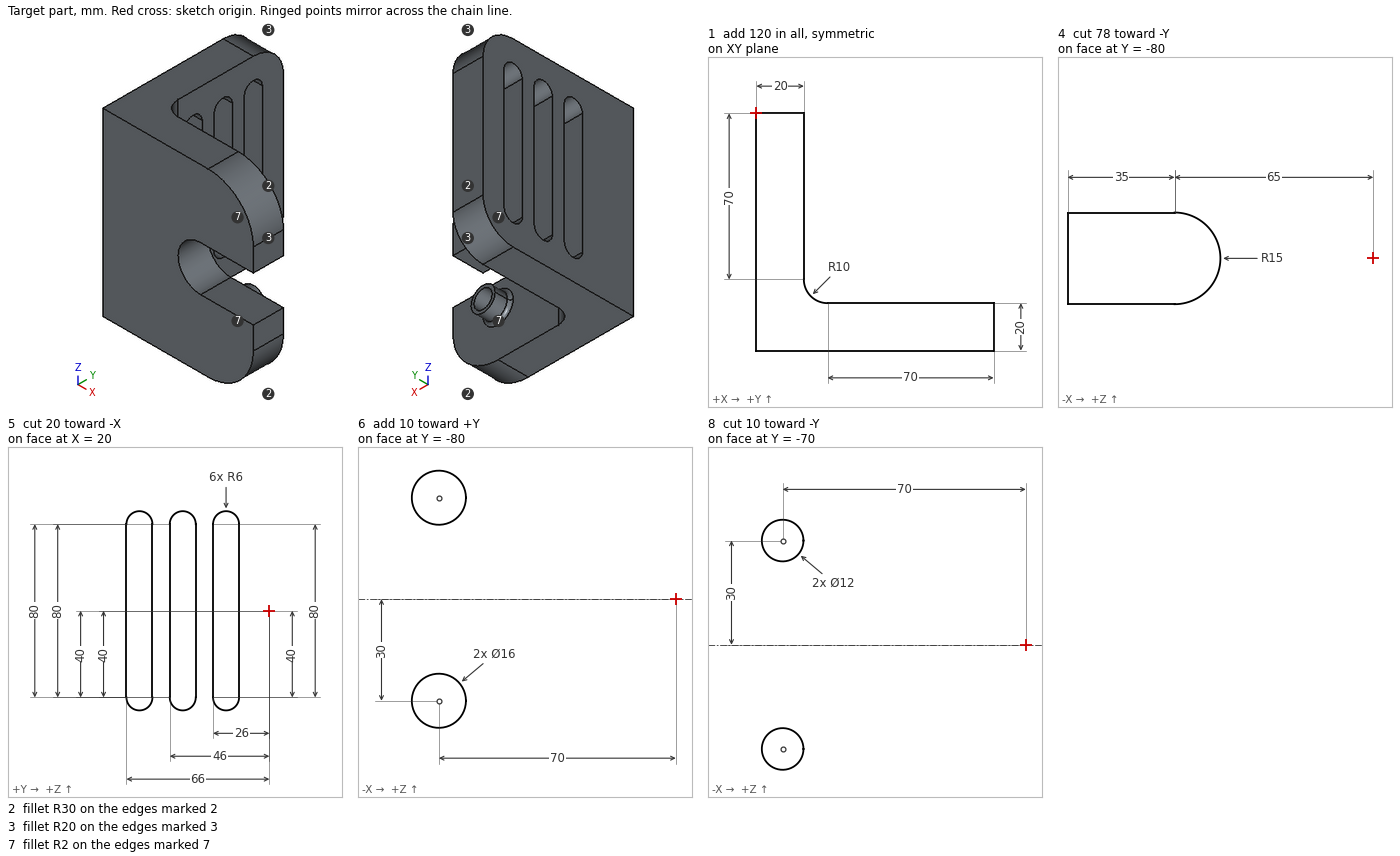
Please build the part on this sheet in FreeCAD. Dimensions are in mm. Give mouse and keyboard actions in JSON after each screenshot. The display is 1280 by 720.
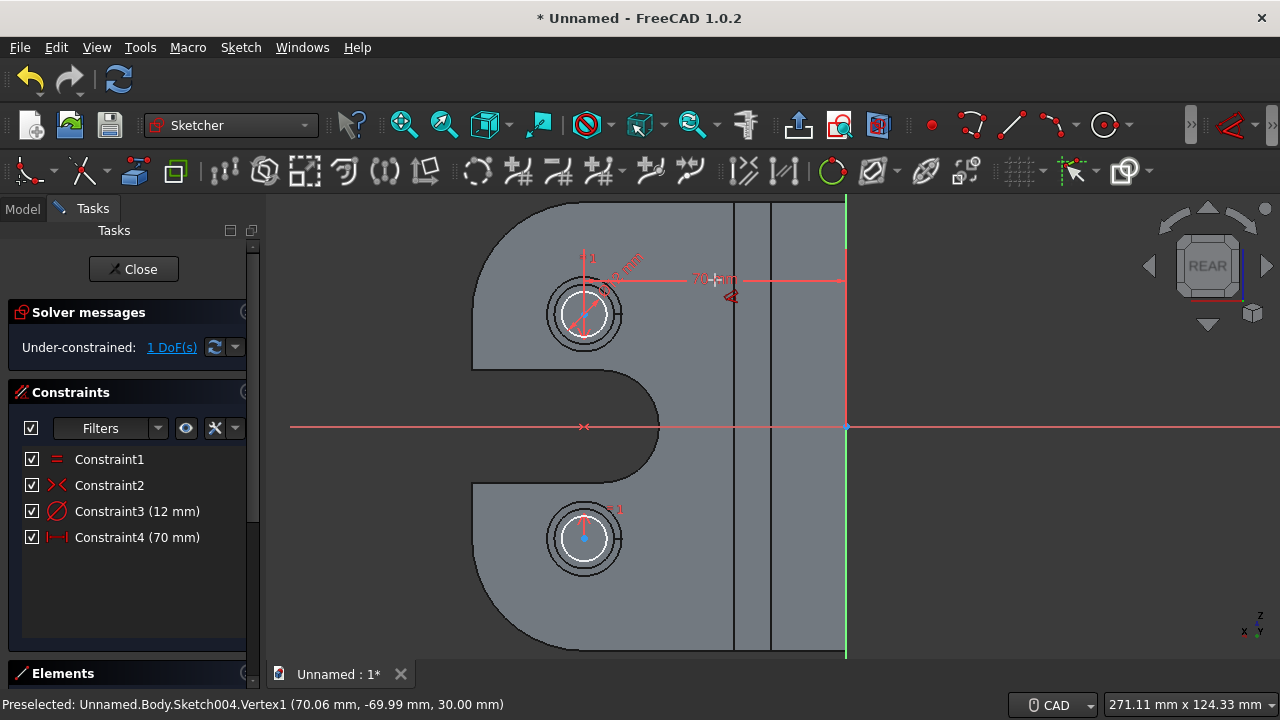
{"action": "left_click", "coordinate": [584, 314]}
{"action": "left_click", "coordinate": [880, 370]}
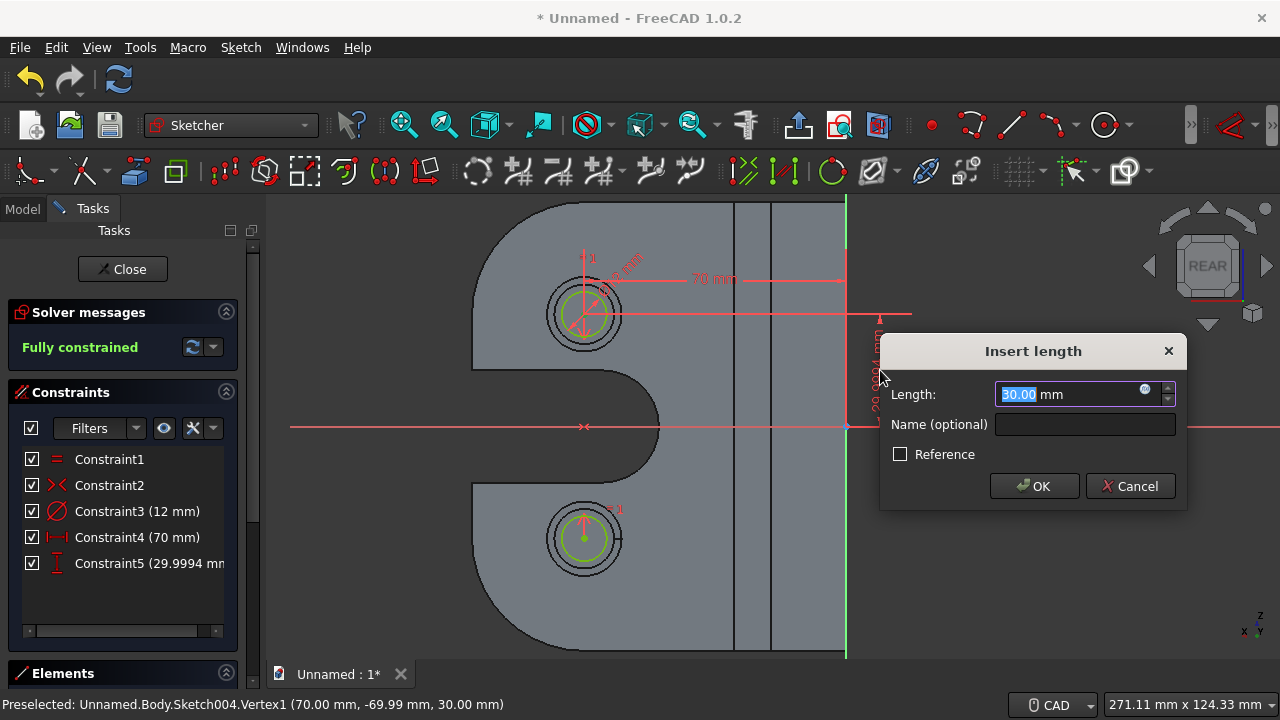
{"action": "type", "text": "30"}
{"action": "key", "text": "Return"}
{"action": "key", "text": "Escape"}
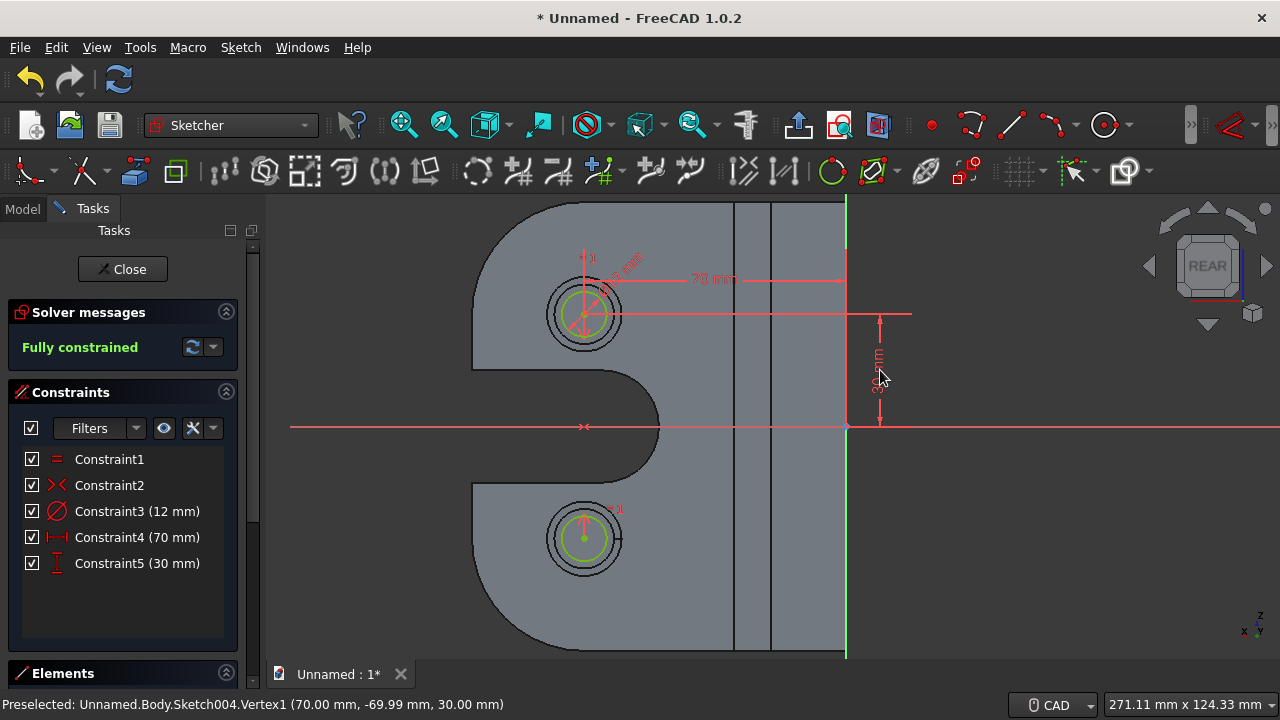
{"action": "left_click", "coordinate": [123, 269]}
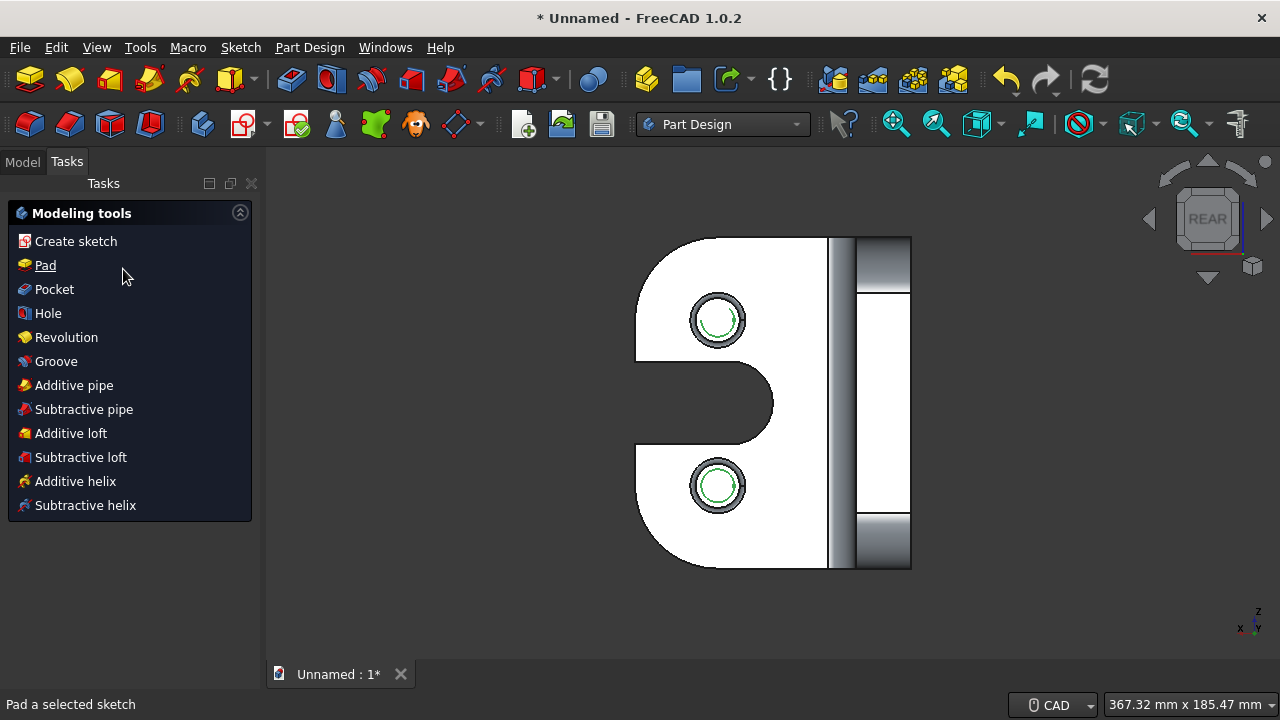
{"action": "left_click", "coordinate": [292, 80]}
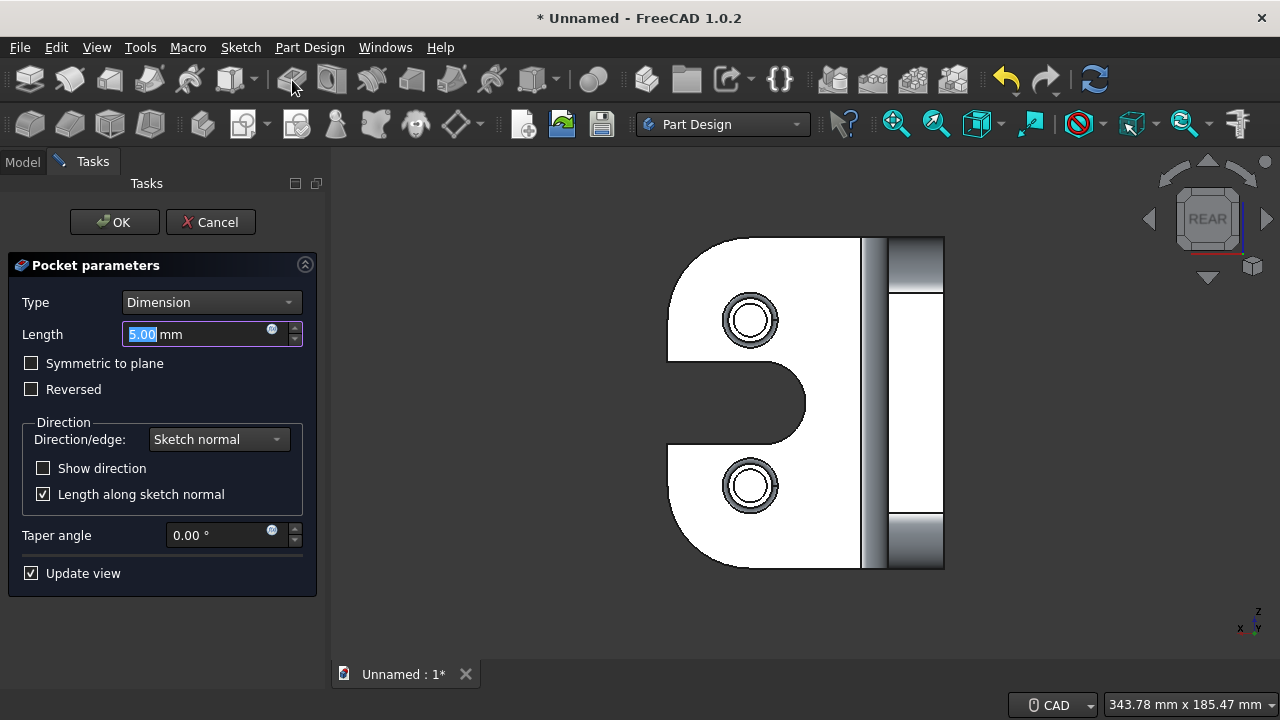
{"action": "type", "text": "10"}
{"action": "key", "text": "Tab"}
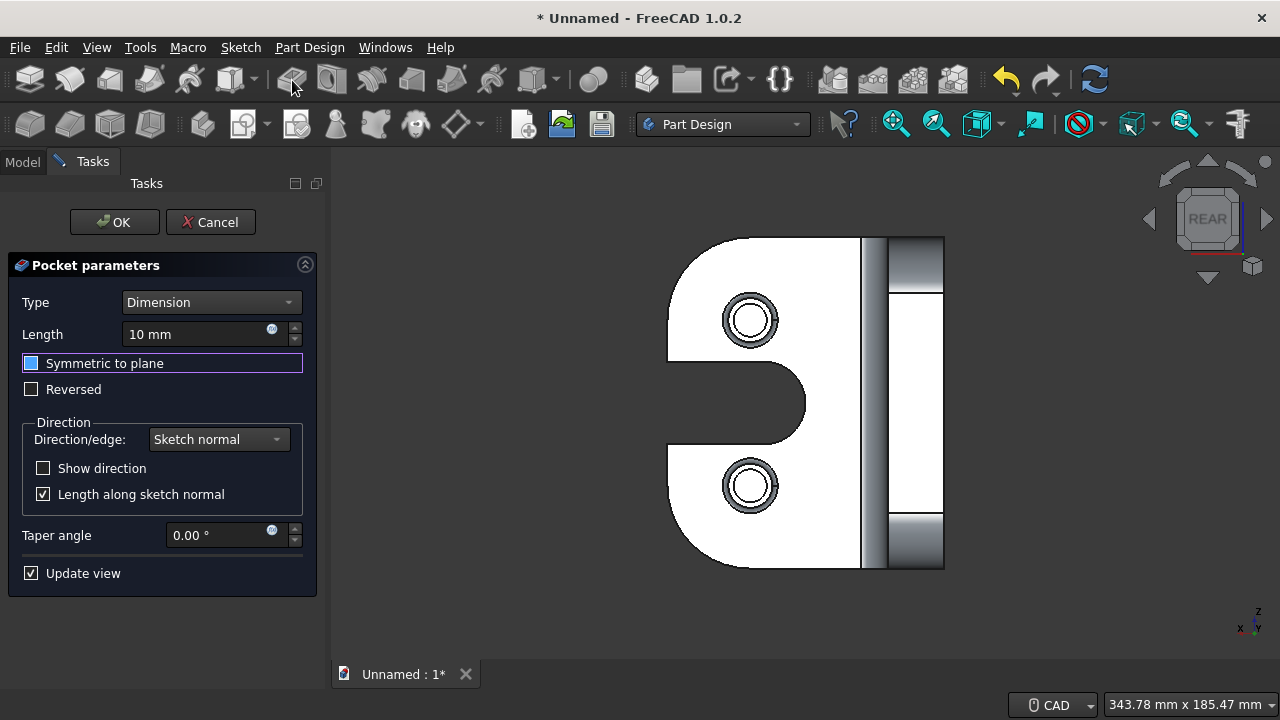
{"action": "left_click", "coordinate": [115, 222]}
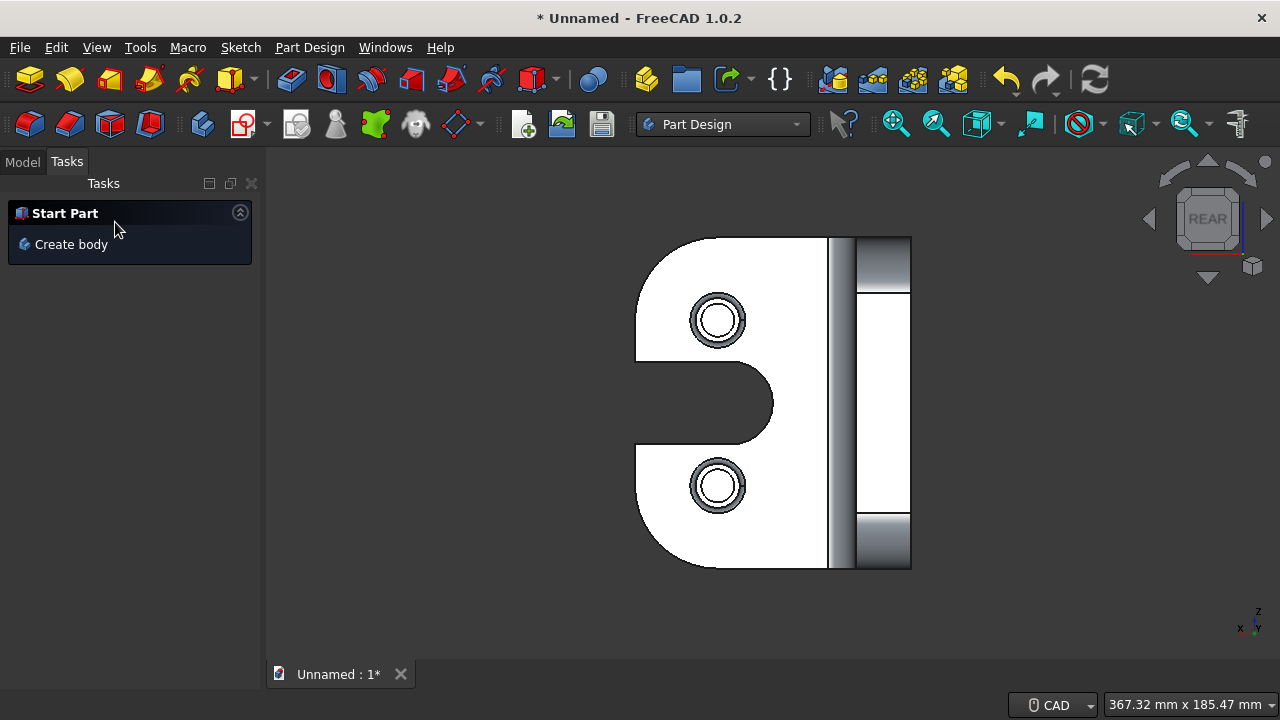
{"action": "key", "text": "0"}